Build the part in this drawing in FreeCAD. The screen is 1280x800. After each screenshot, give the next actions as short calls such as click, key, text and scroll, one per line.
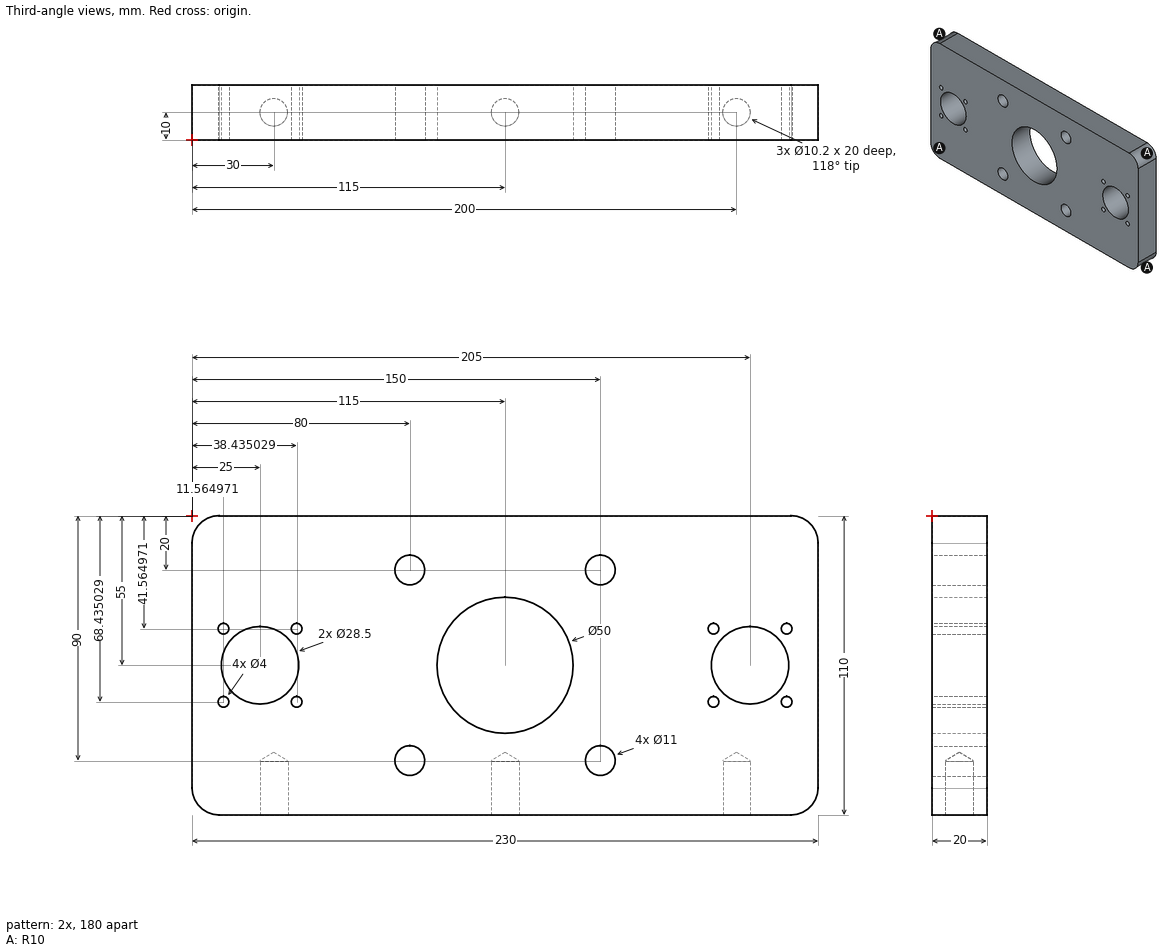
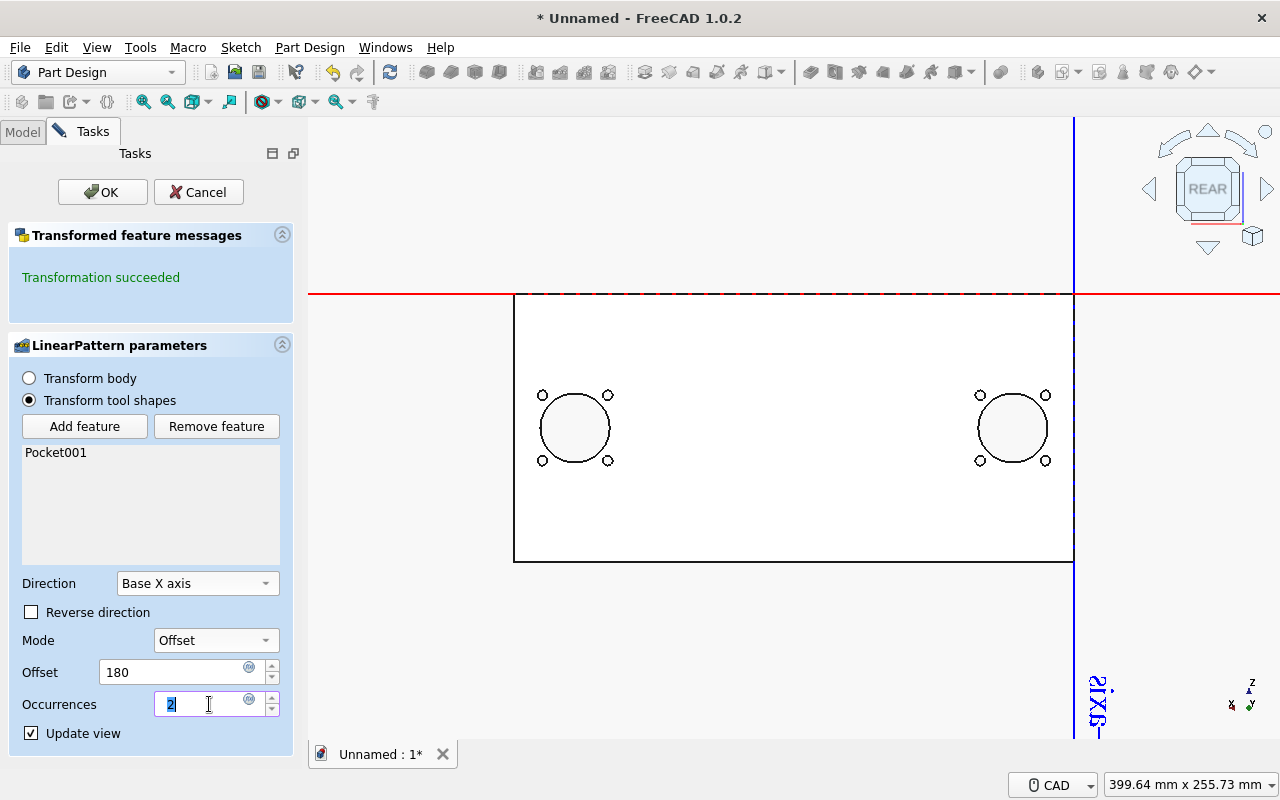
text(2)
key(Tab)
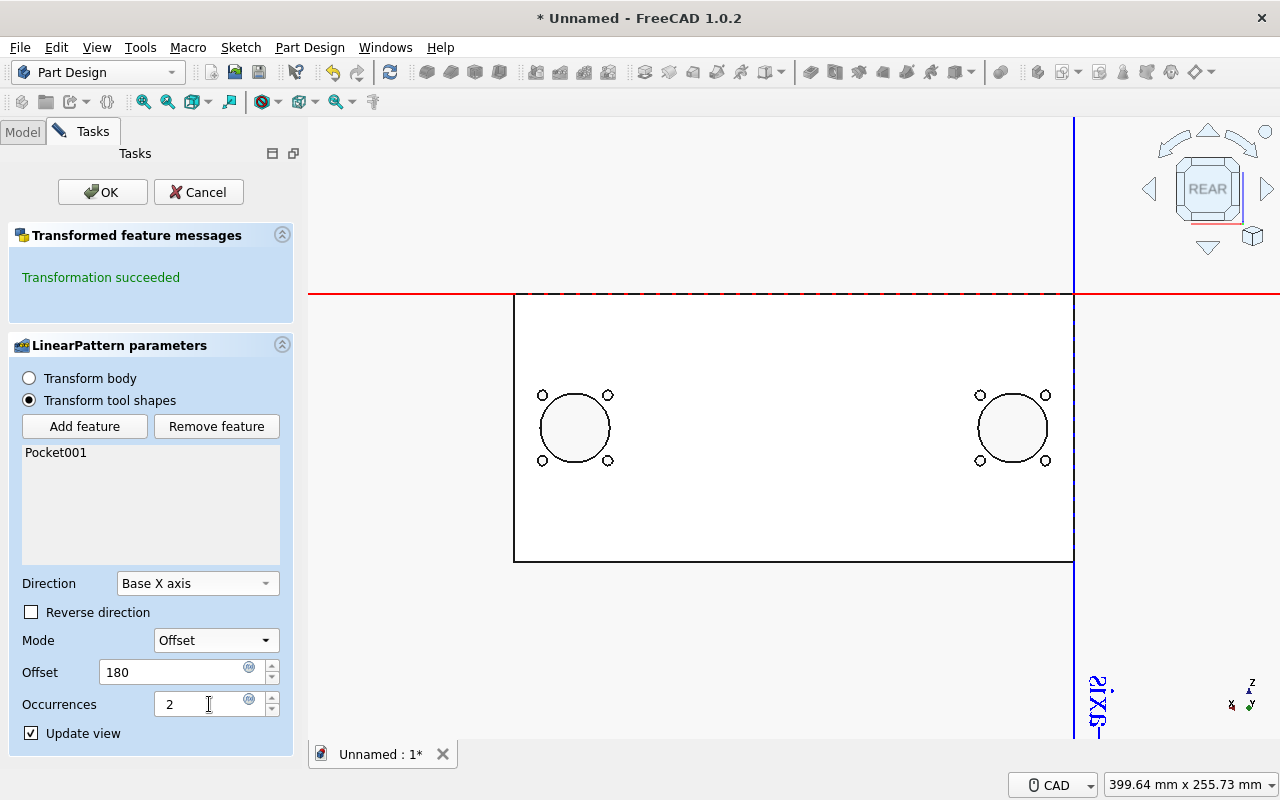
click(103, 192)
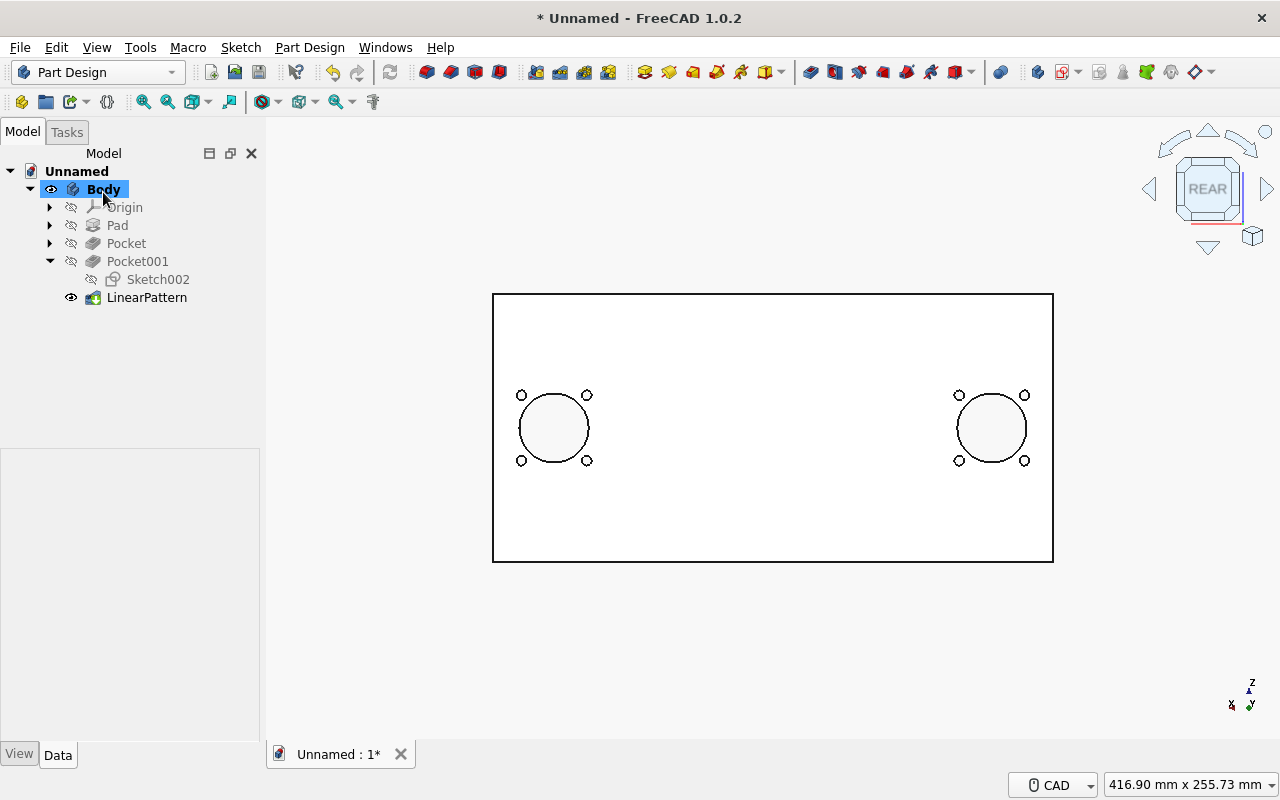
key(0)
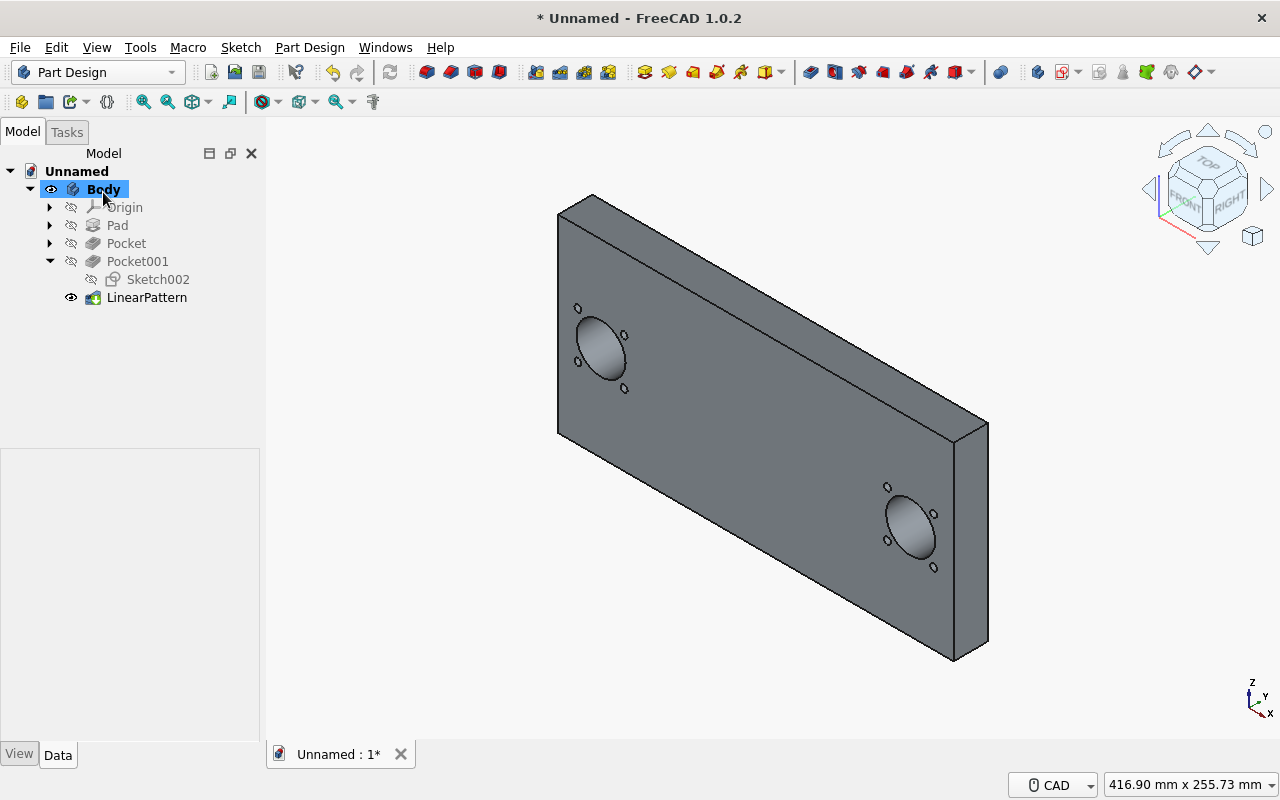
click(971, 432)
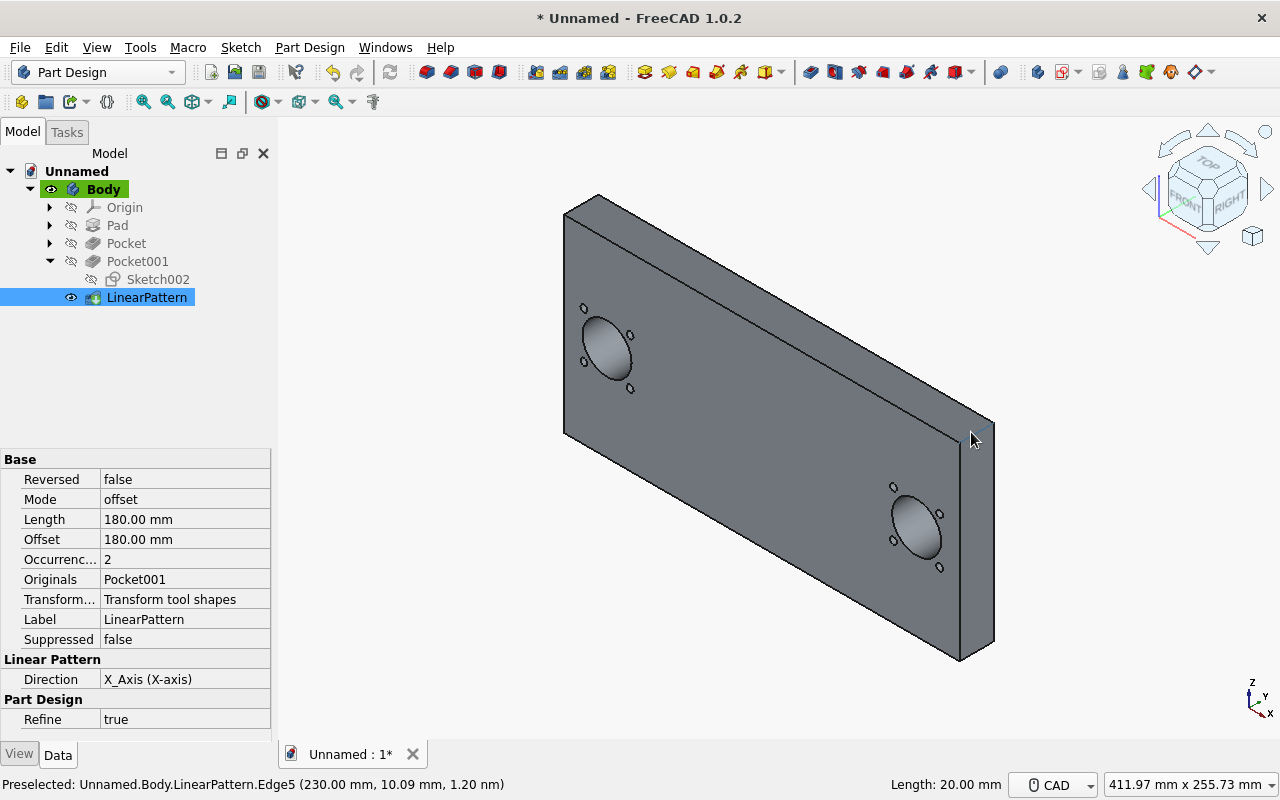
key(2)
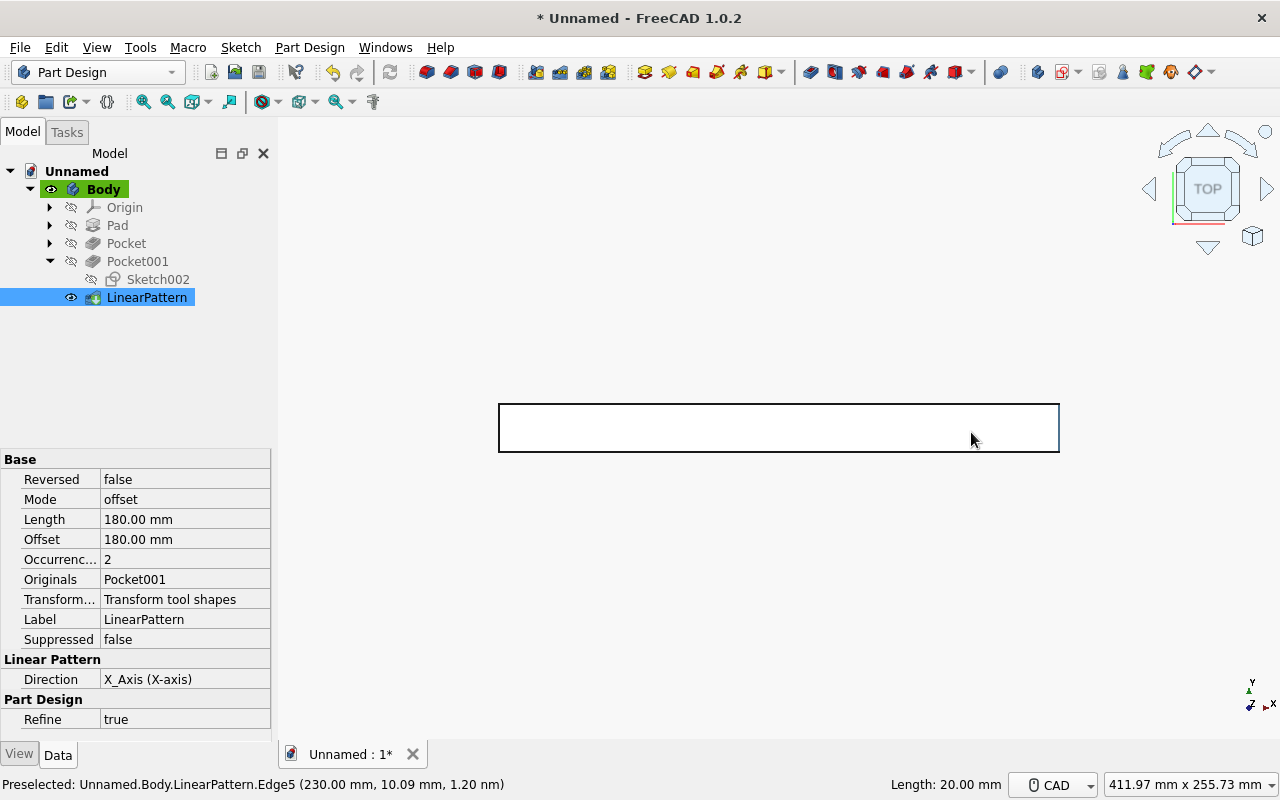
click(499, 427, ctrl)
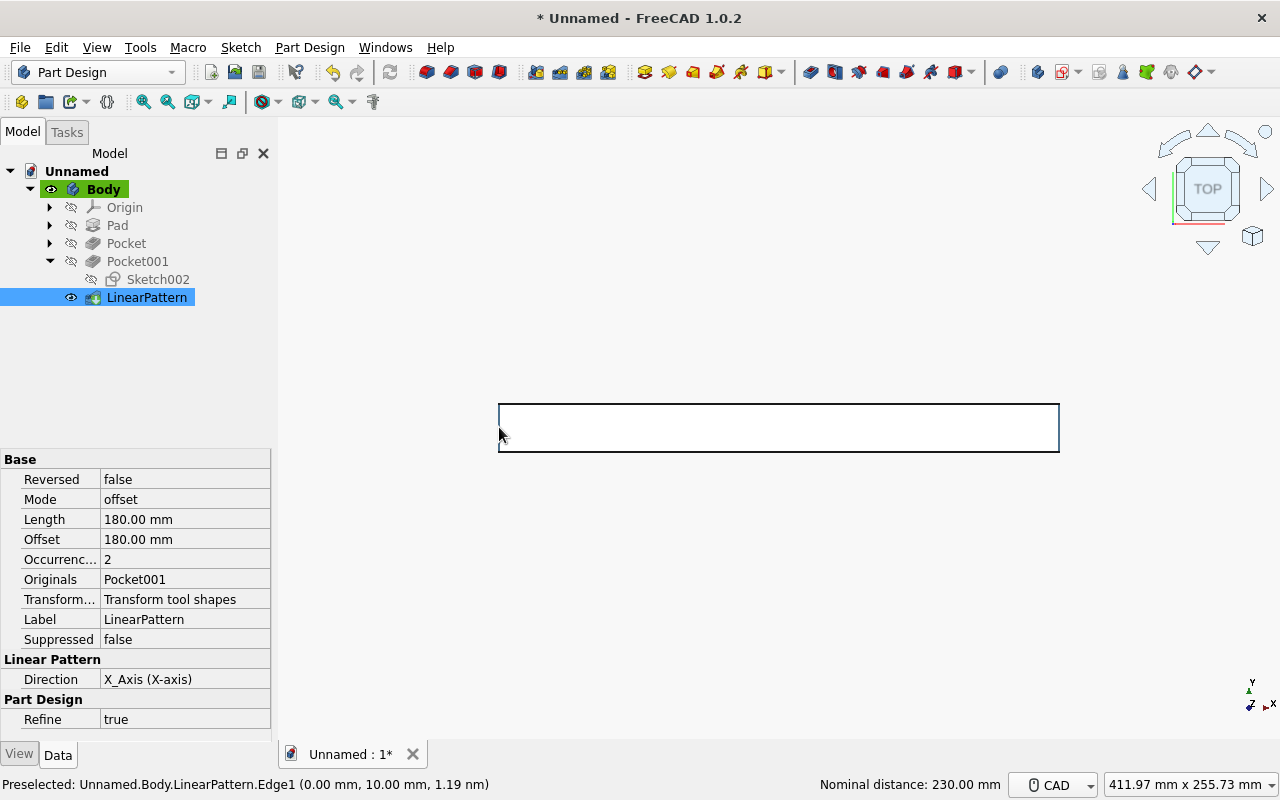
key(1)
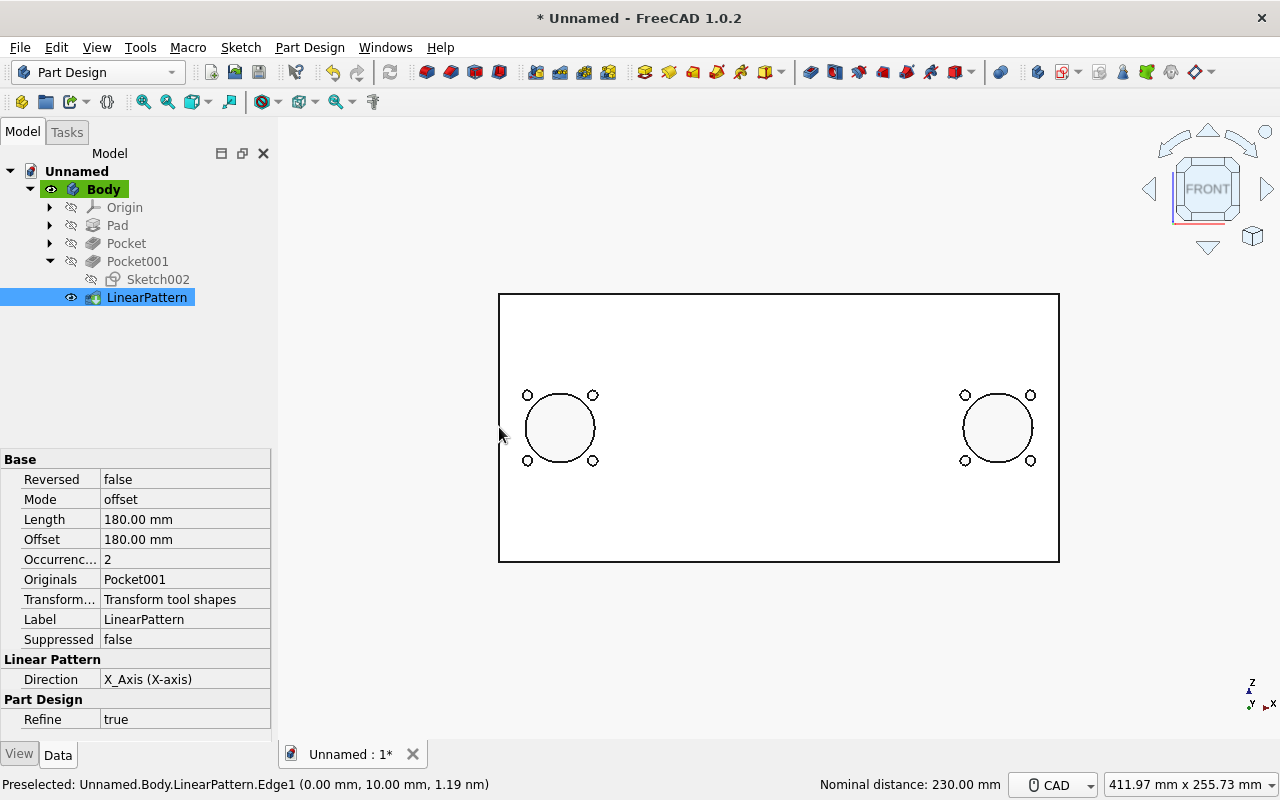
key(3)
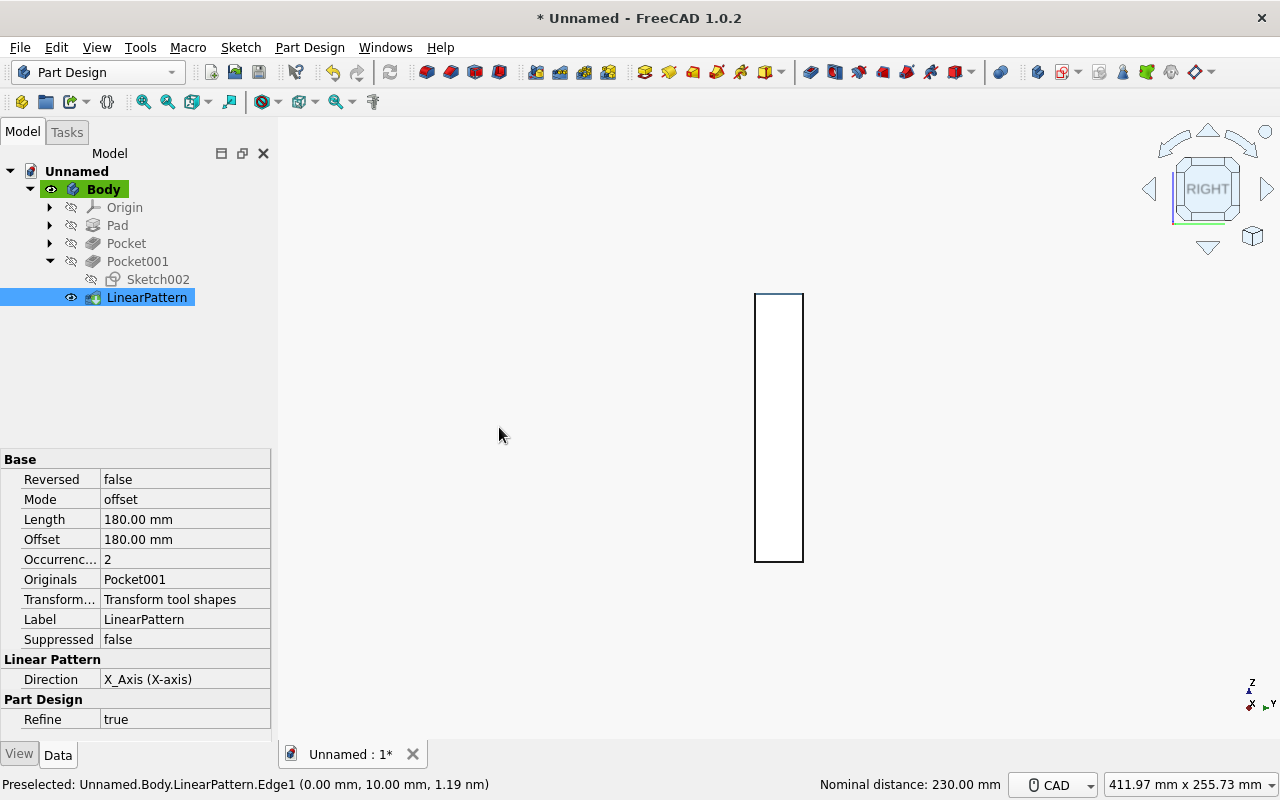
key(v)
key(f)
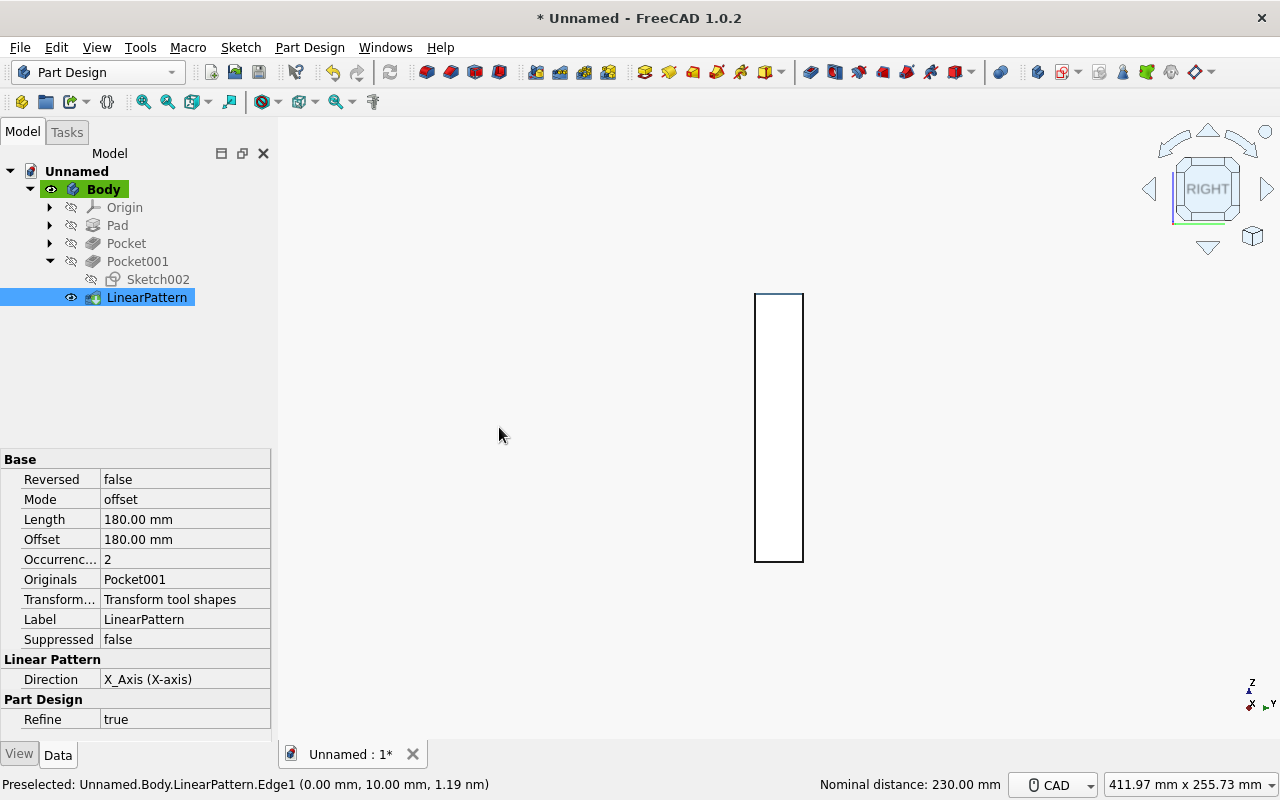
click(779, 561, ctrl)